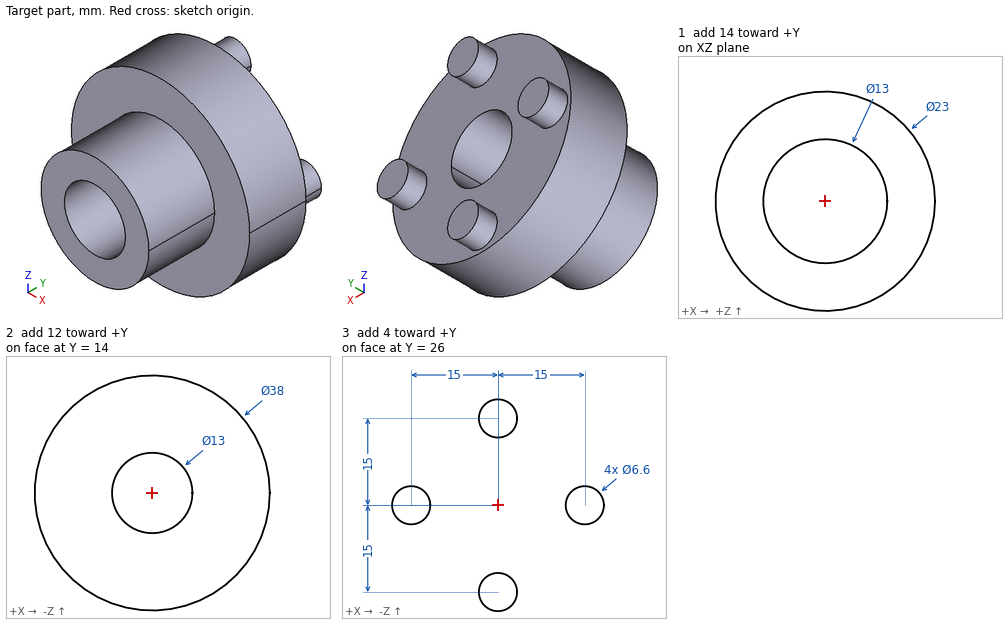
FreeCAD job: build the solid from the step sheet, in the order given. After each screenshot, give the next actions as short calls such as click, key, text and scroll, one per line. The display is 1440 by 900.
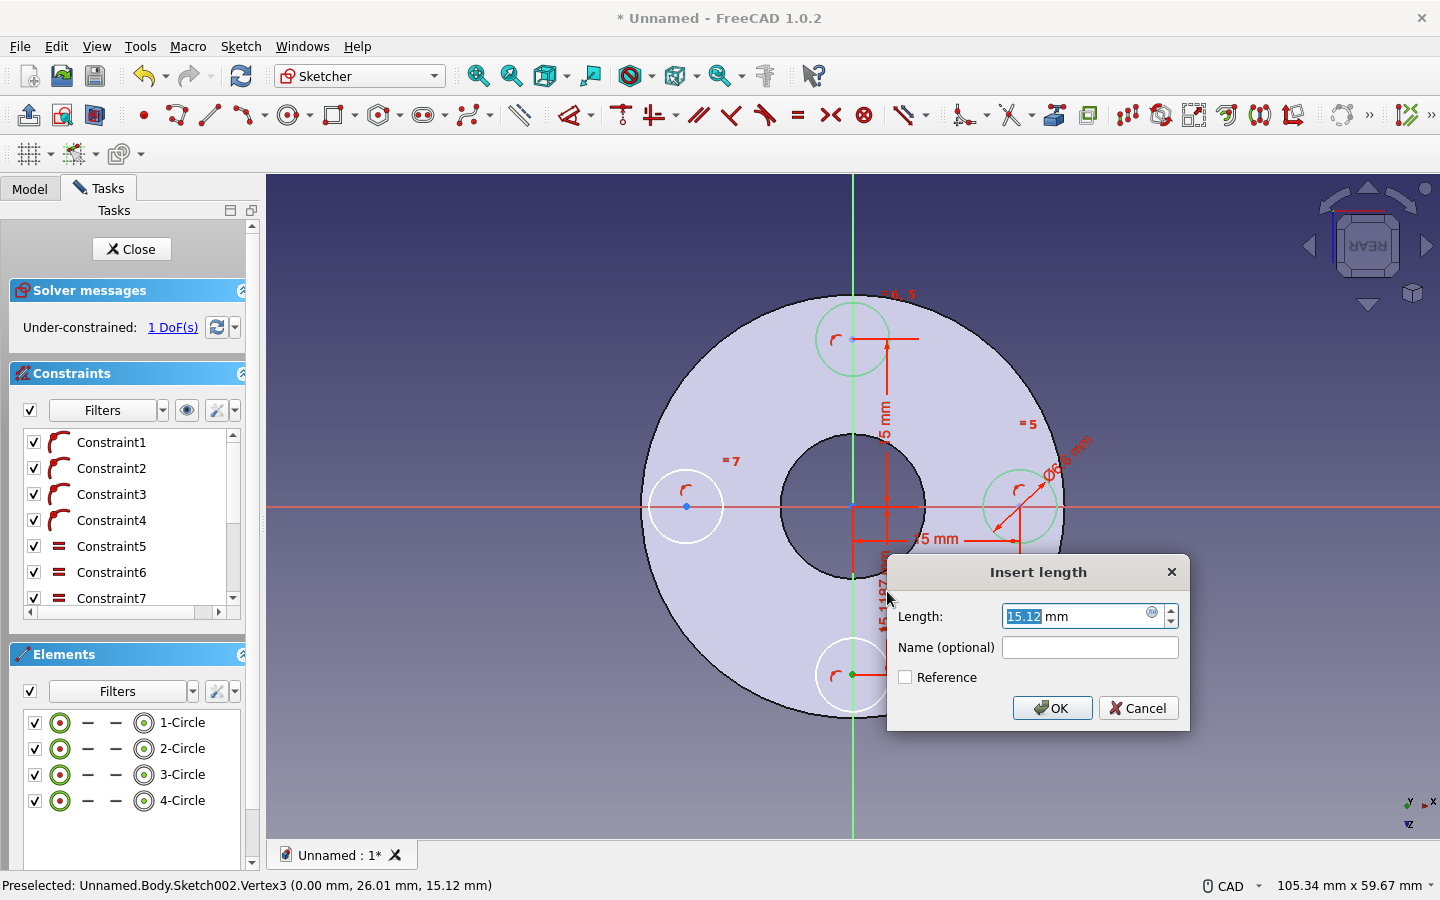
text(15)
key(Return)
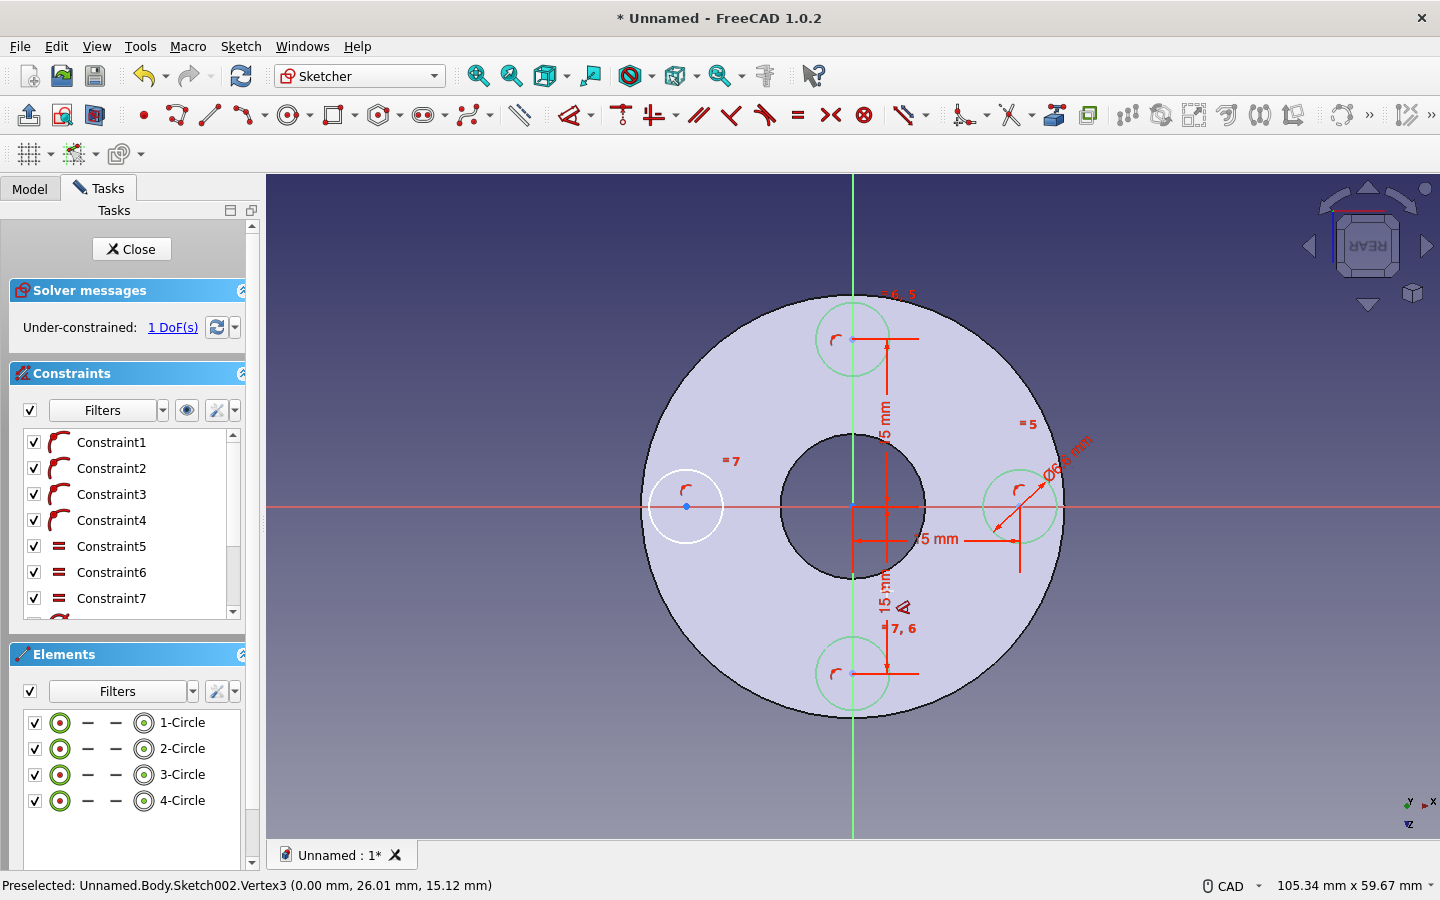
click(686, 506)
click(769, 540)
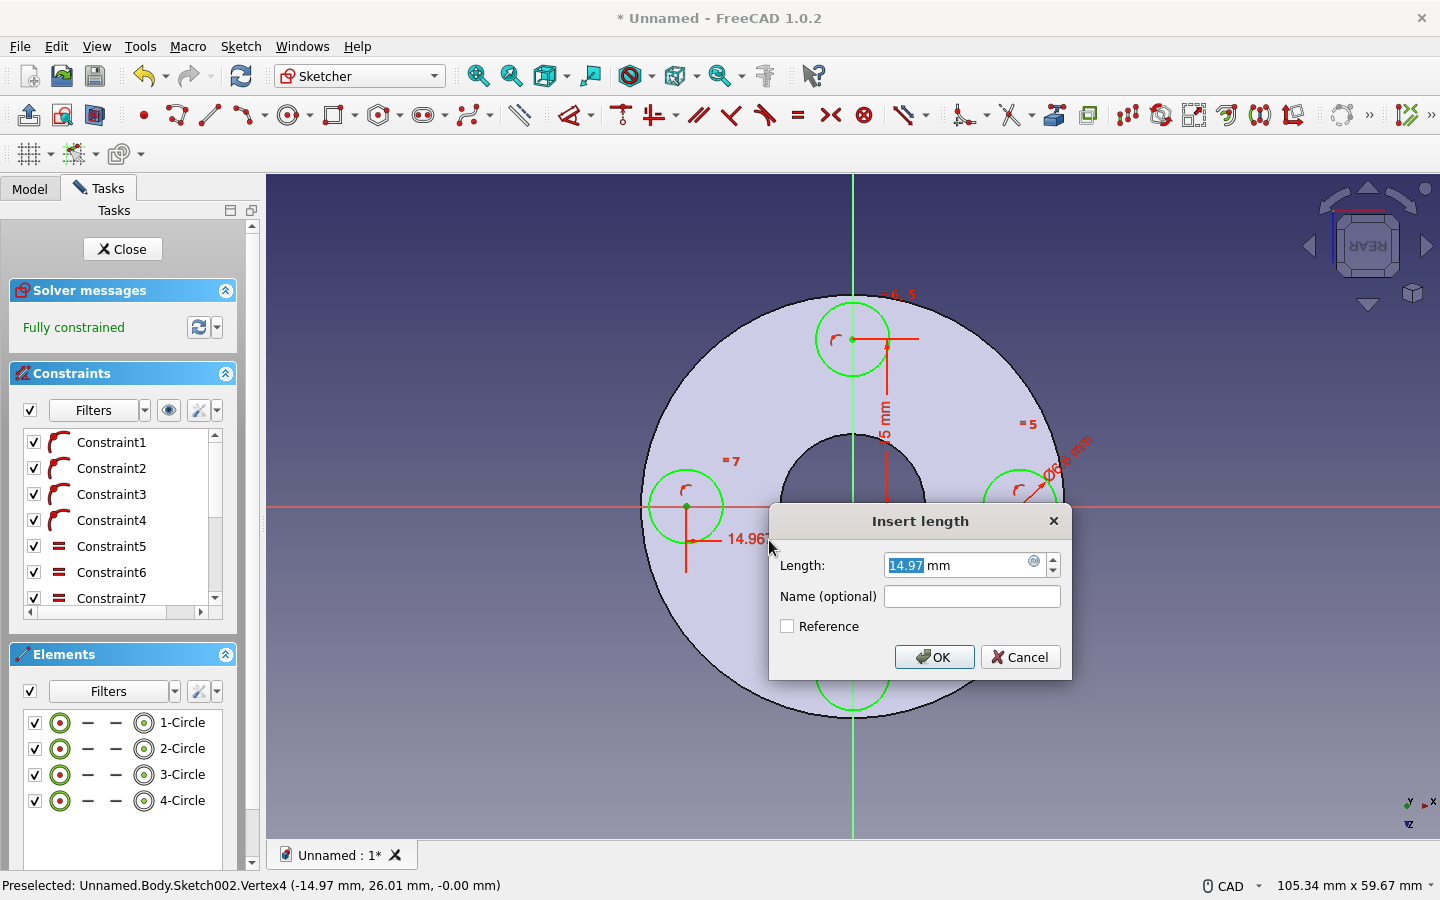
text(15)
key(Return)
key(Escape)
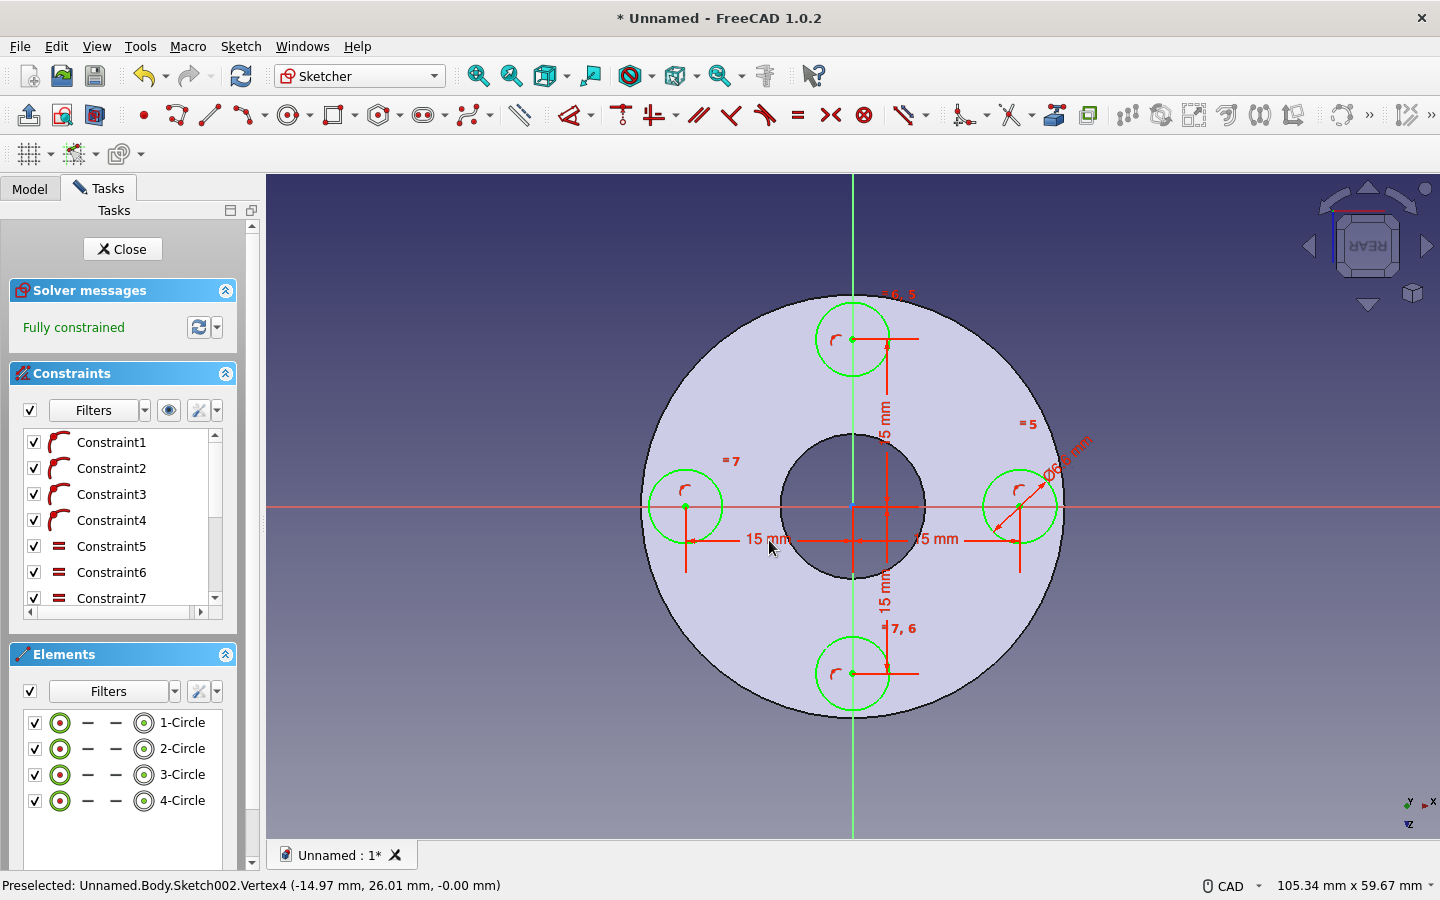
click(123, 249)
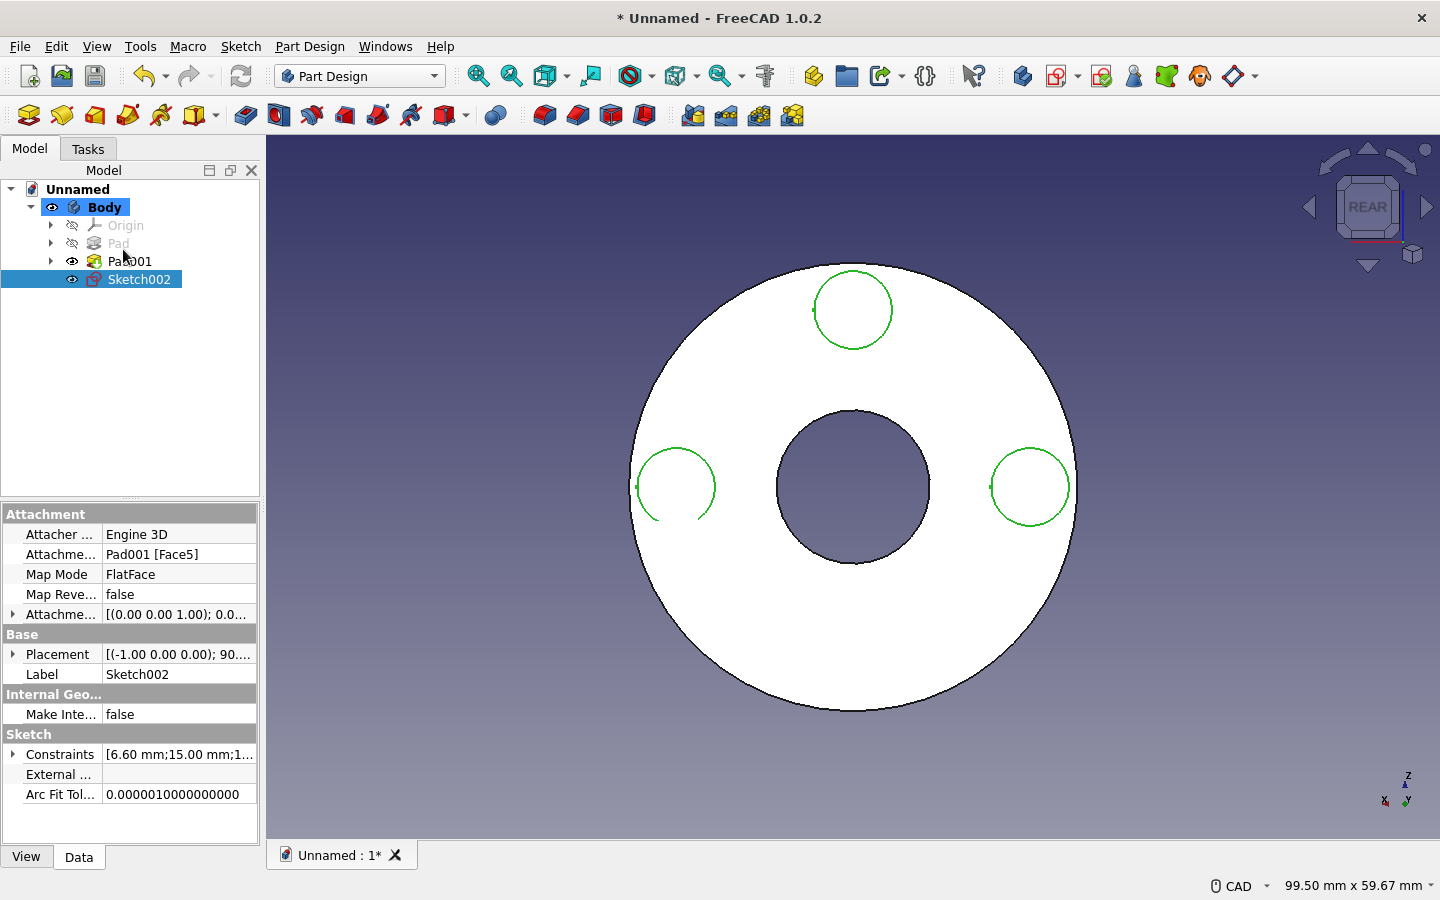
click(29, 116)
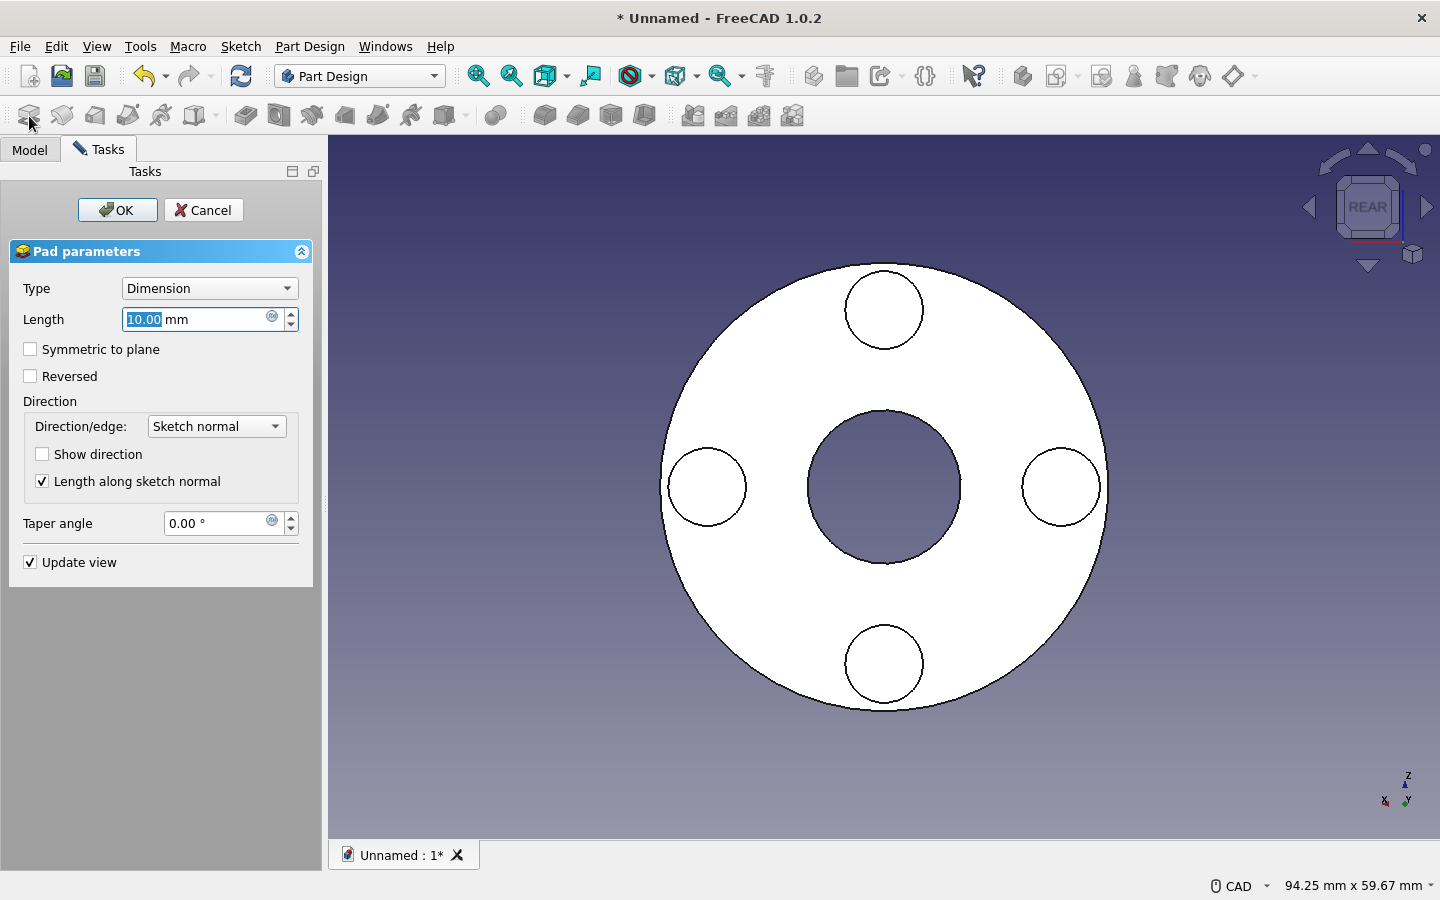
text(4)
key(Tab)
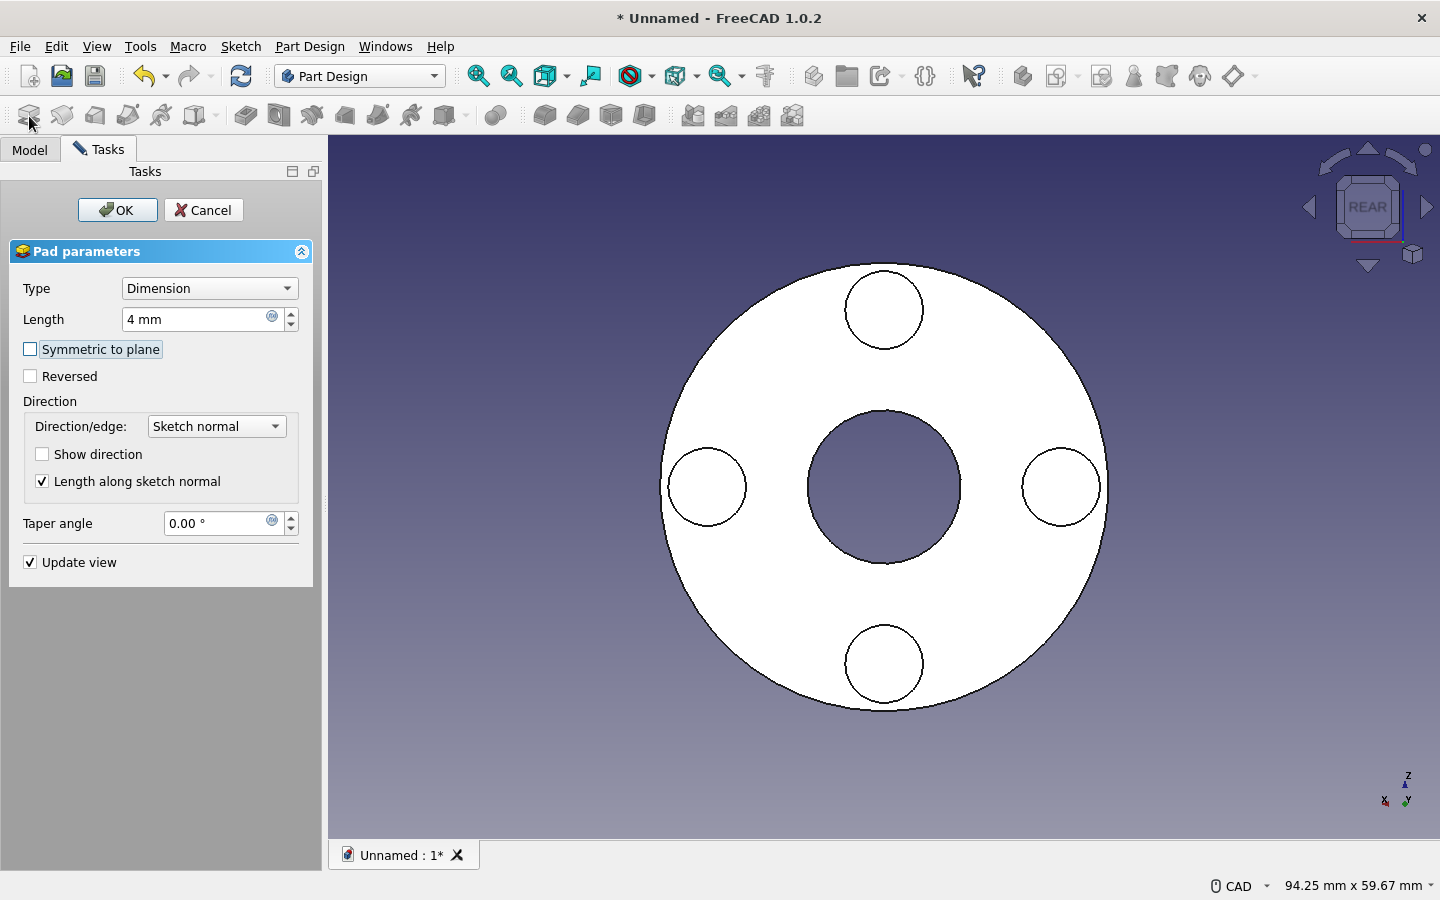
click(118, 210)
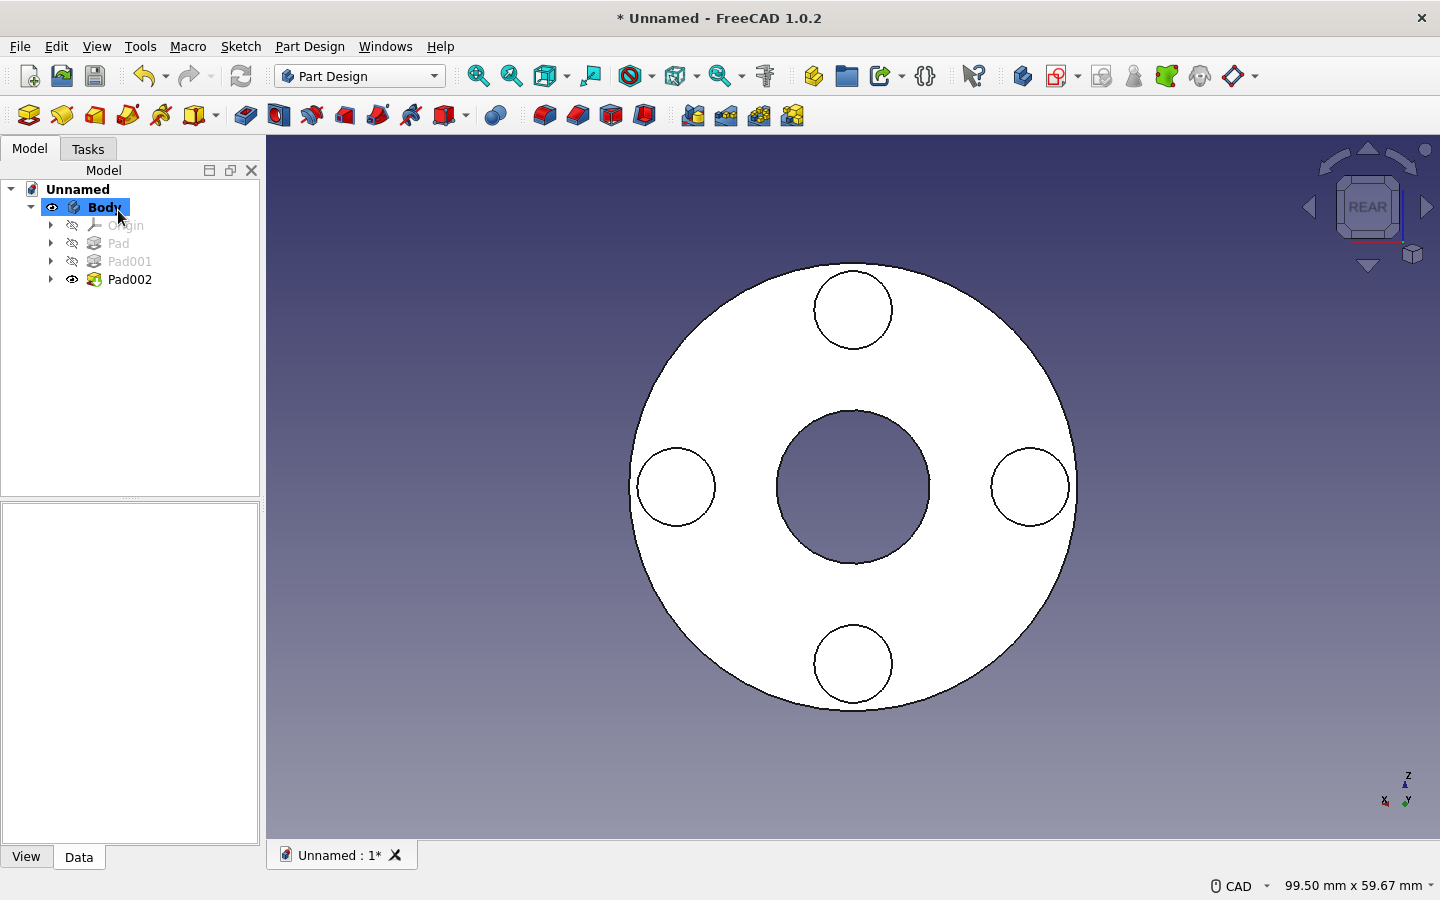
key(0)